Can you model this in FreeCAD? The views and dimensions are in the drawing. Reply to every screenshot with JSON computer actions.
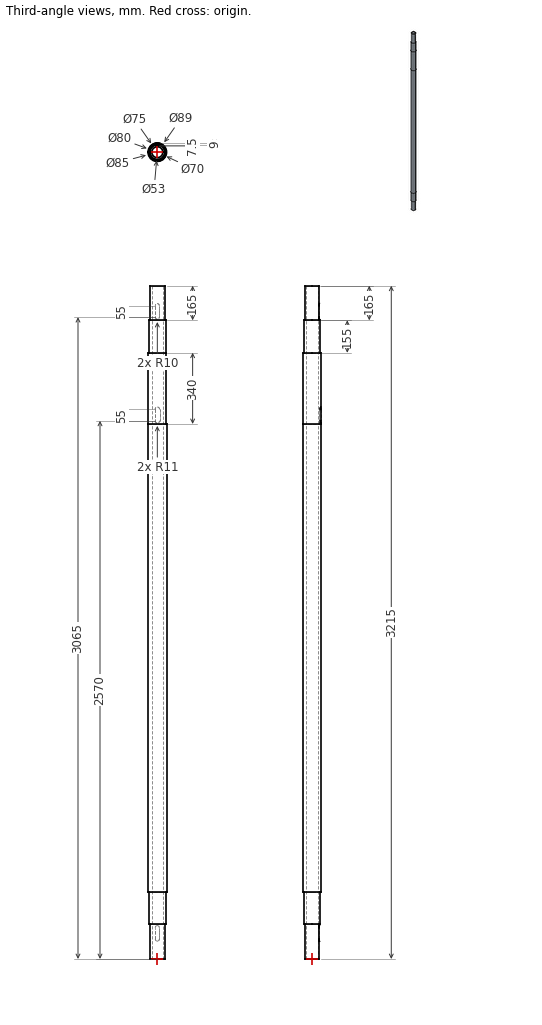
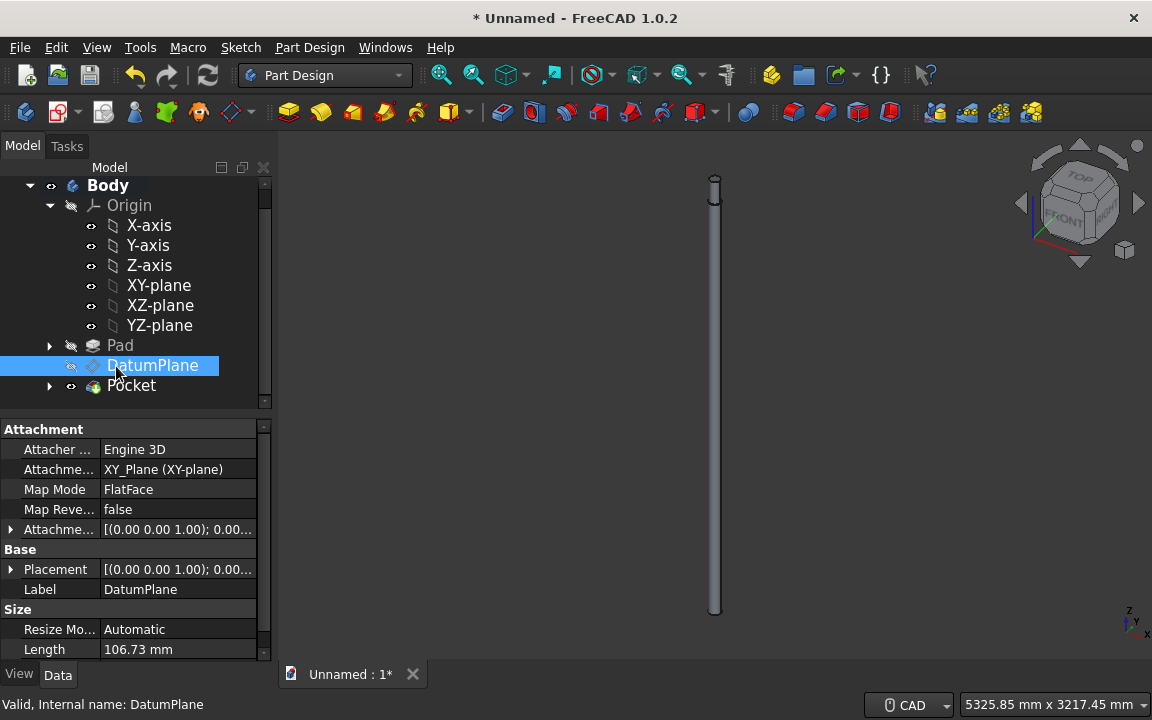
{"action": "left_click", "coordinate": [136, 286]}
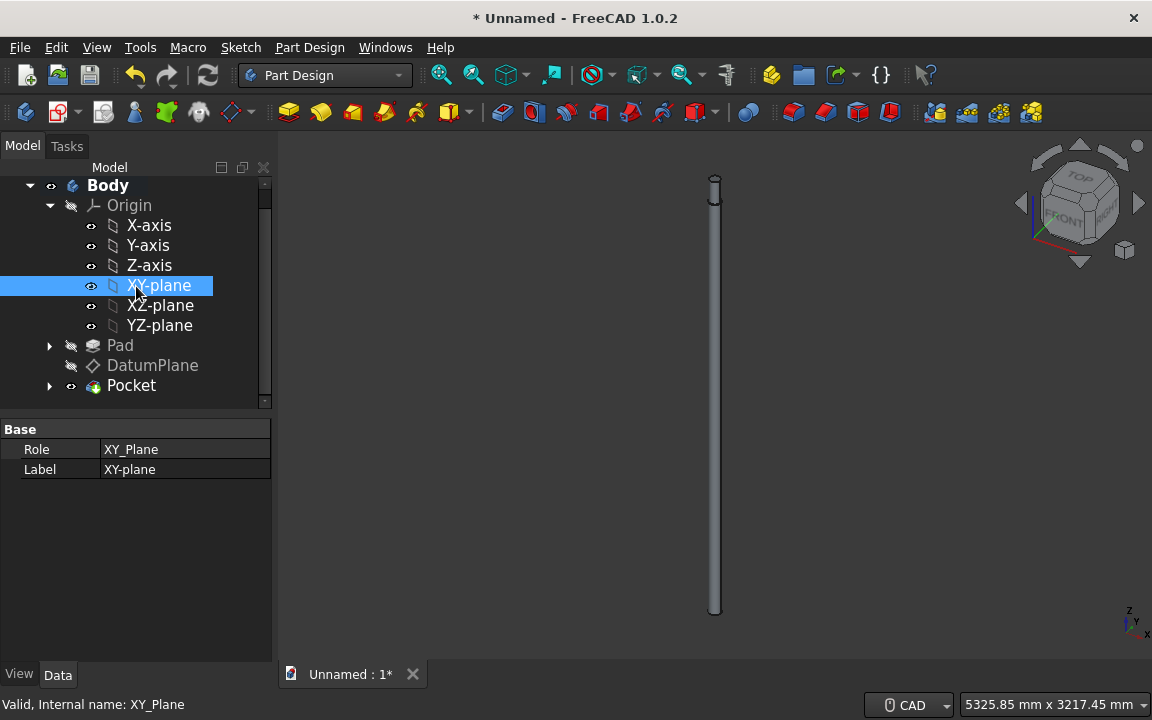
{"action": "left_click", "coordinate": [232, 112]}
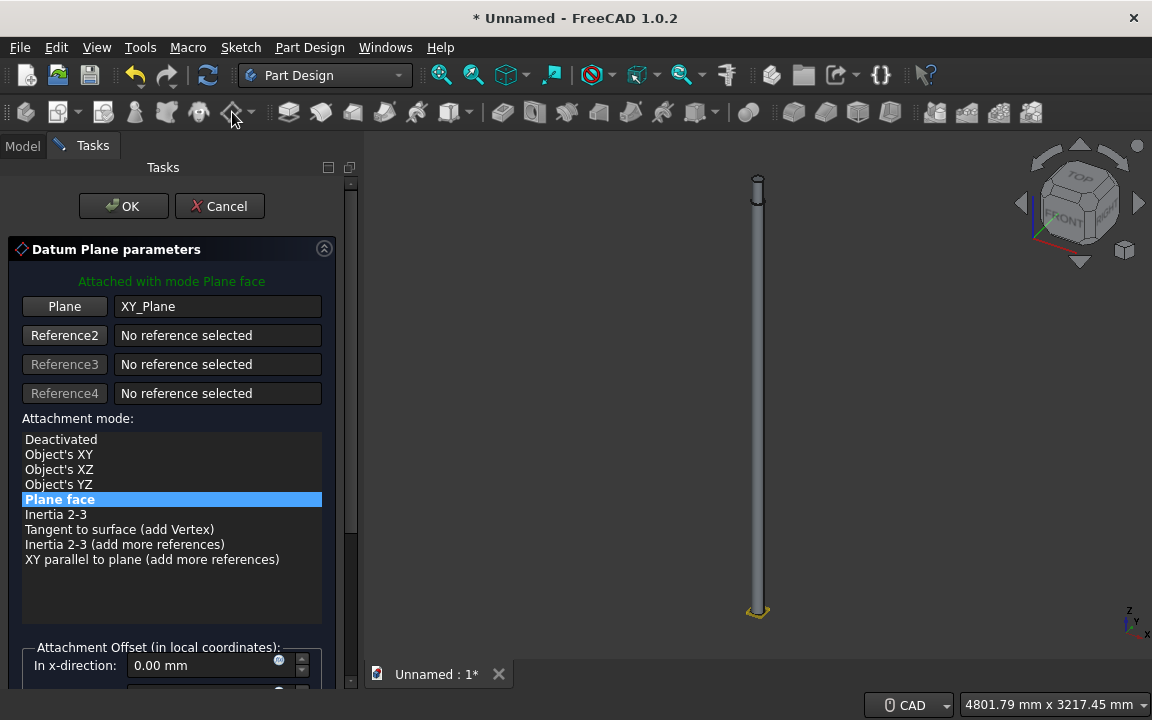
{"action": "scroll", "coordinate": [351, 432], "scroll_direction": "down", "scroll_amount": 2}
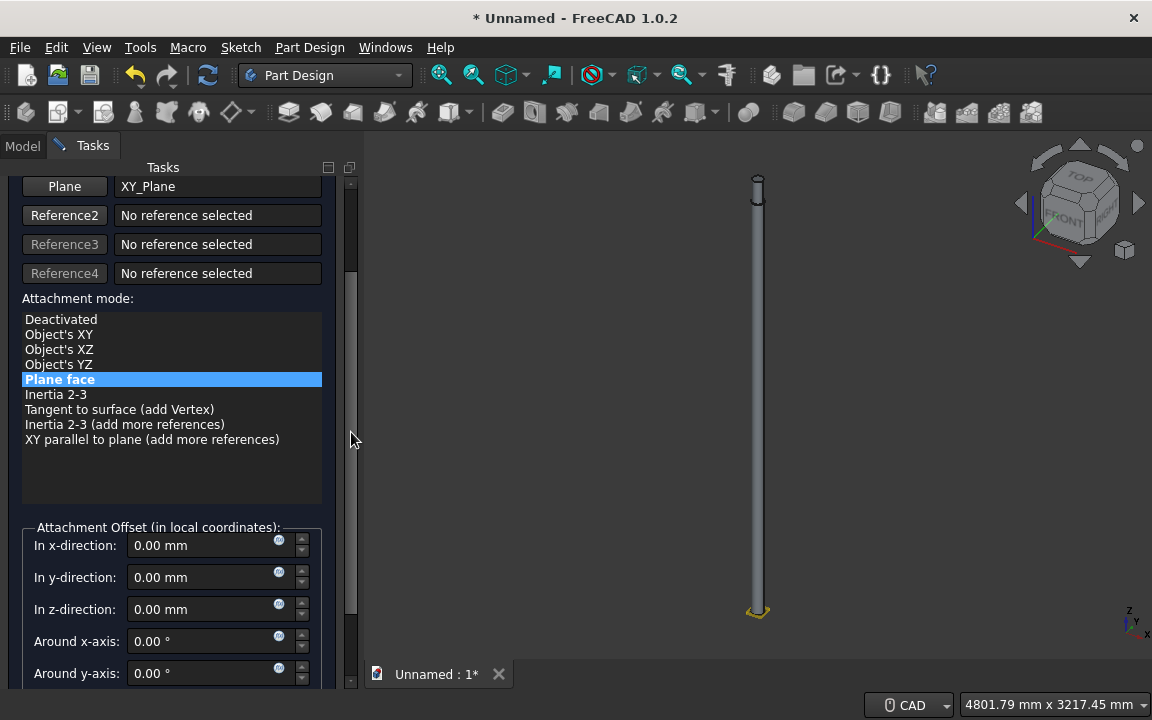
{"action": "triple_click", "coordinate": [210, 609]}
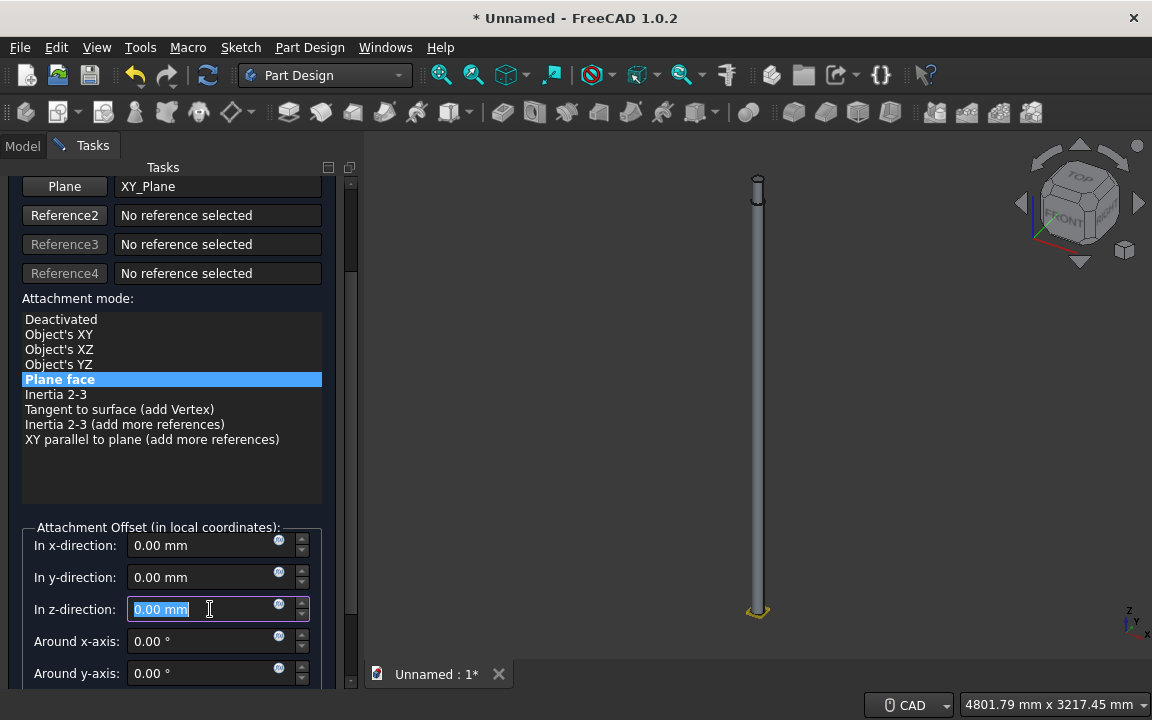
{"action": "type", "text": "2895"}
{"action": "key", "text": "Tab"}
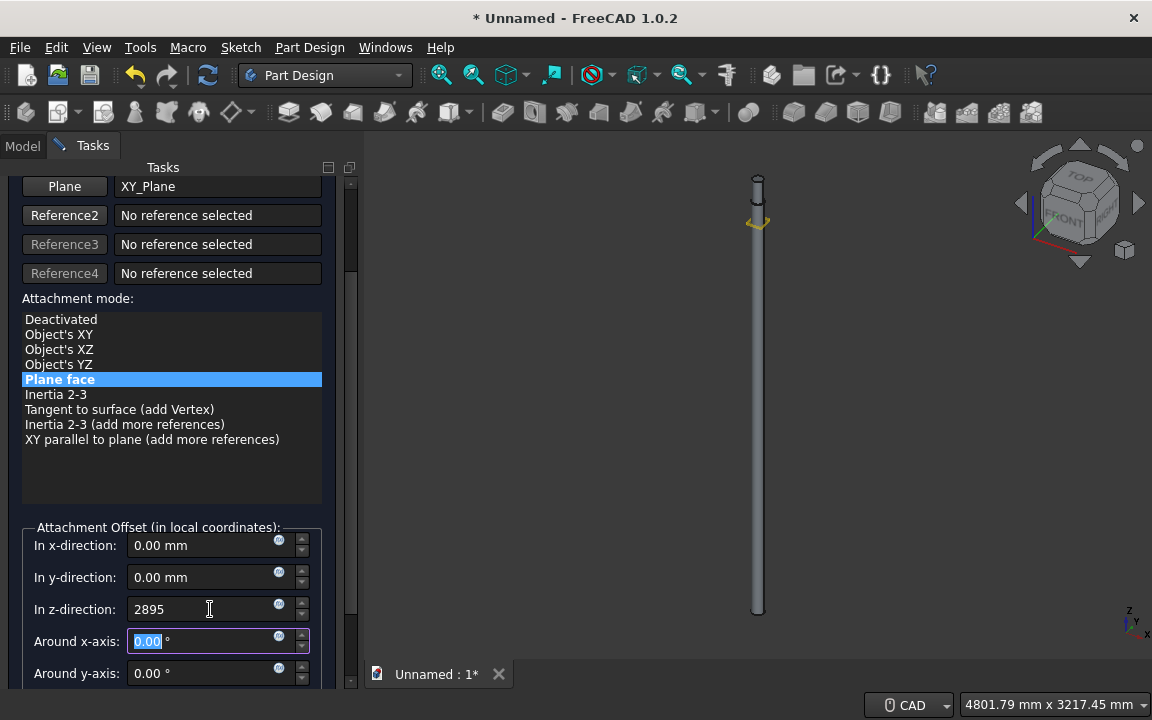
{"action": "scroll", "coordinate": [351, 432], "scroll_direction": "up", "scroll_amount": 3}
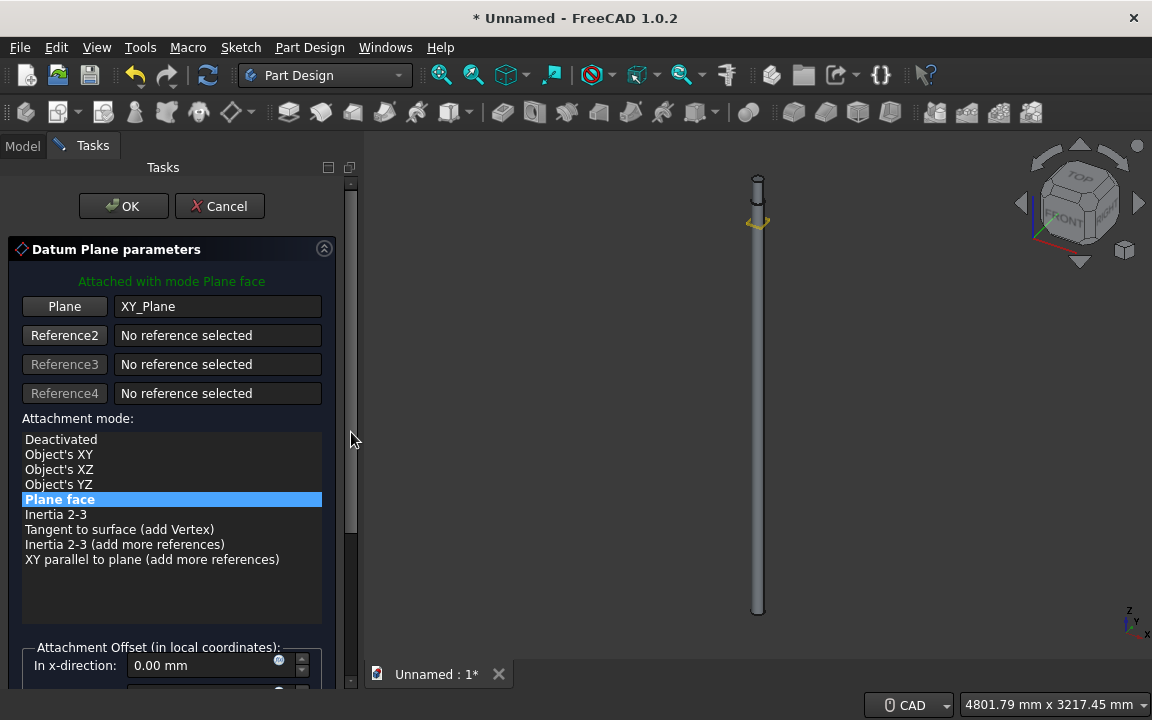
{"action": "left_click", "coordinate": [124, 206]}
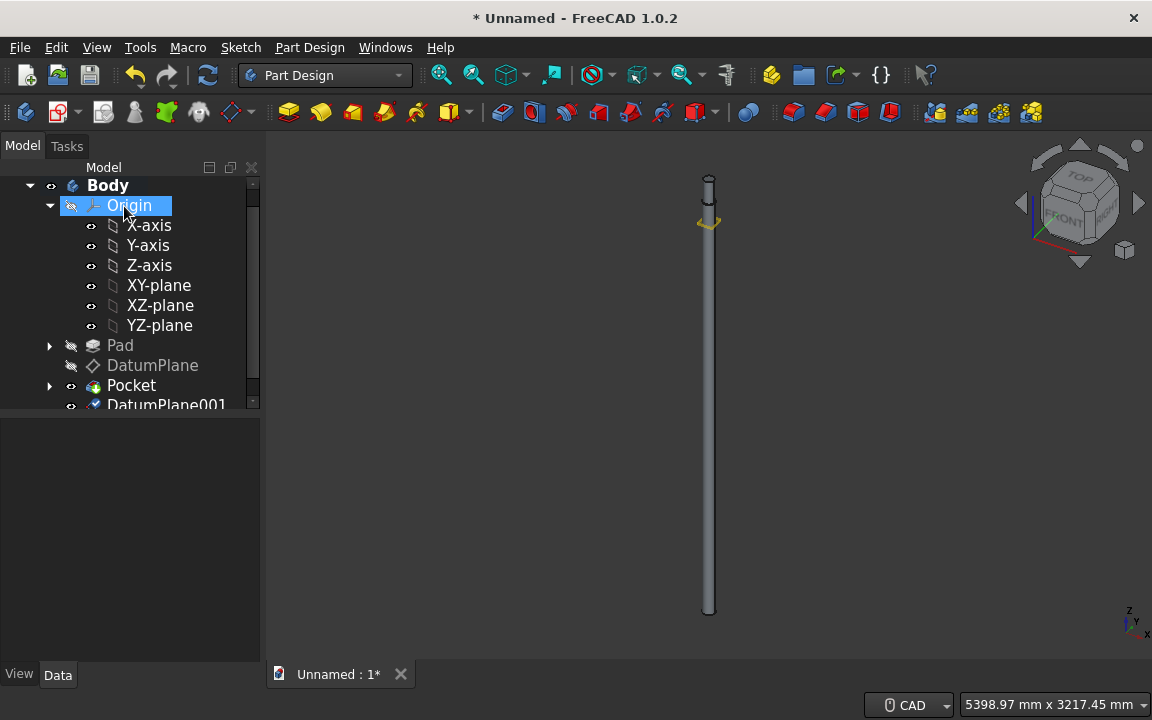
{"action": "left_click", "coordinate": [116, 406]}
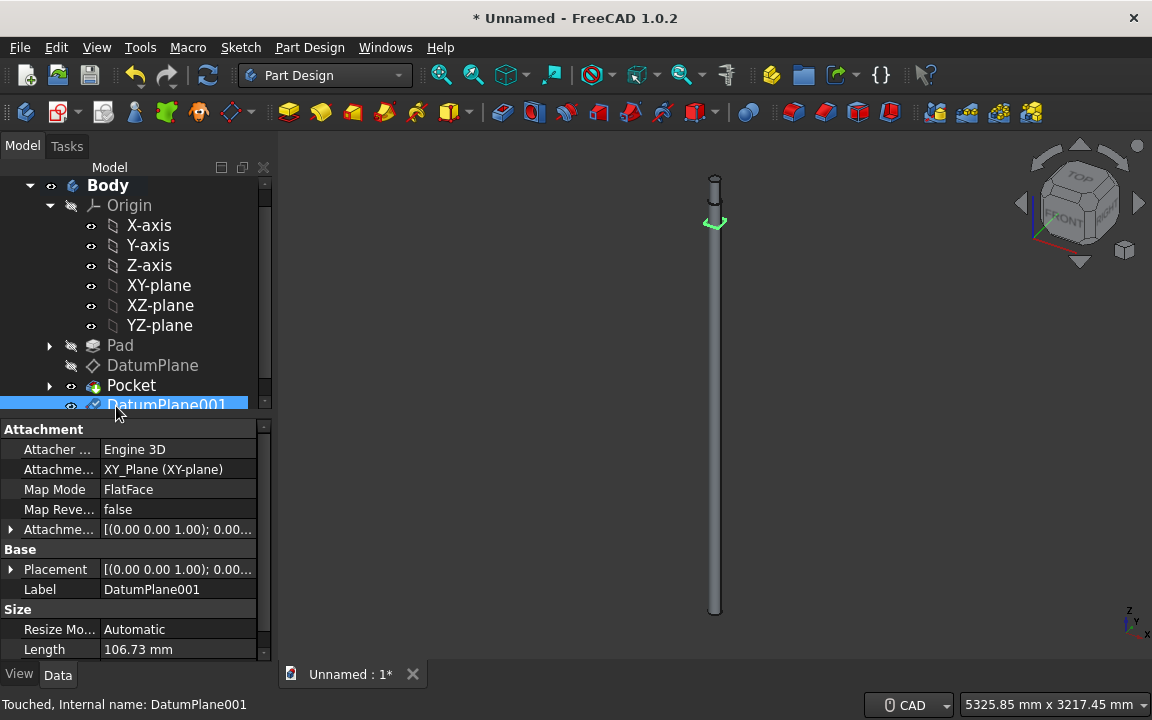
{"action": "left_click", "coordinate": [58, 112]}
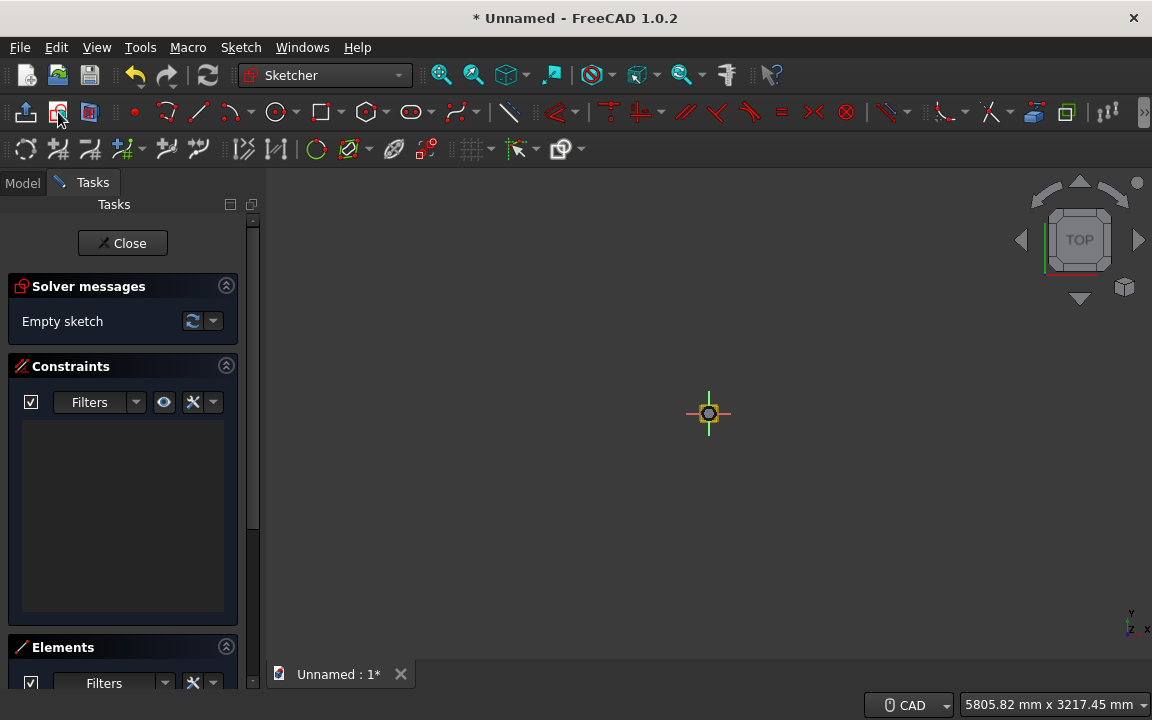
{"action": "left_click", "coordinate": [90, 112]}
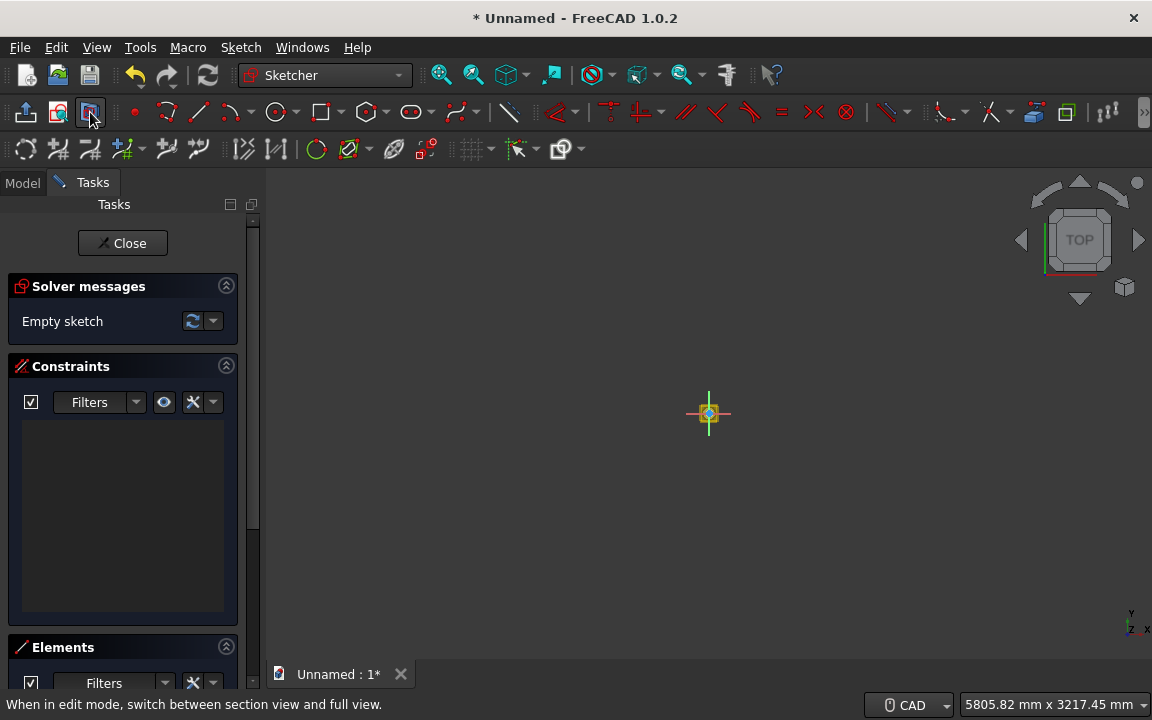
{"action": "scroll", "coordinate": [713, 414], "scroll_direction": "up", "scroll_amount": 15}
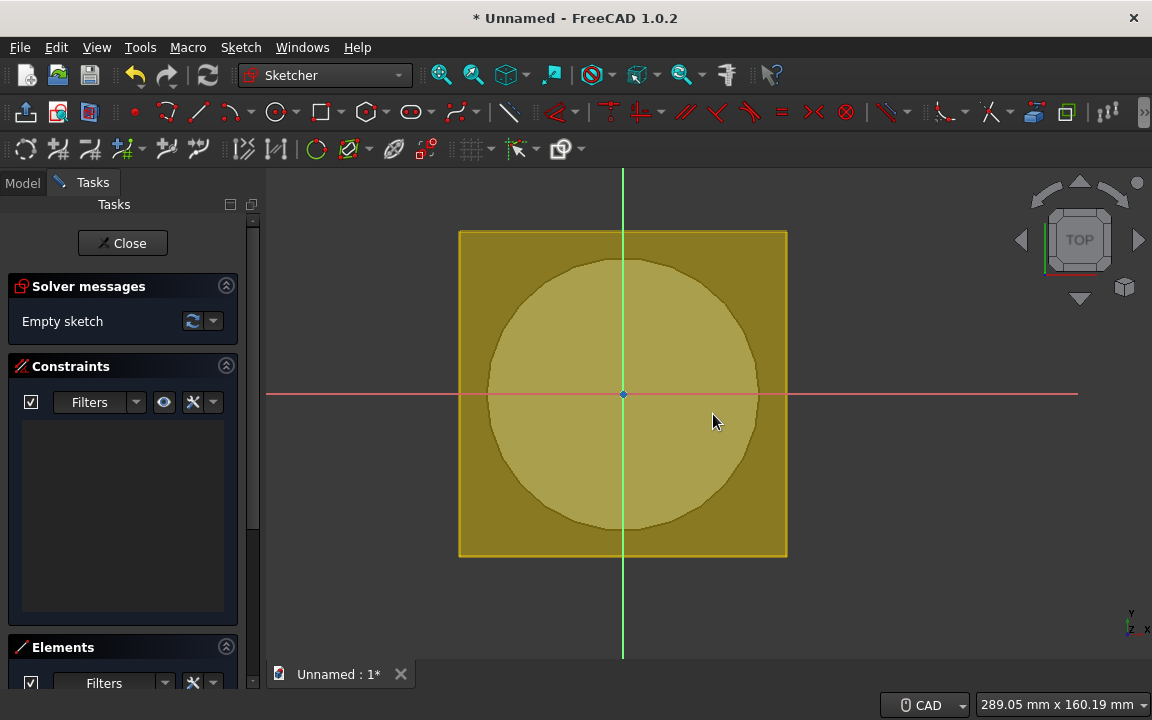
{"action": "left_click", "coordinate": [276, 112]}